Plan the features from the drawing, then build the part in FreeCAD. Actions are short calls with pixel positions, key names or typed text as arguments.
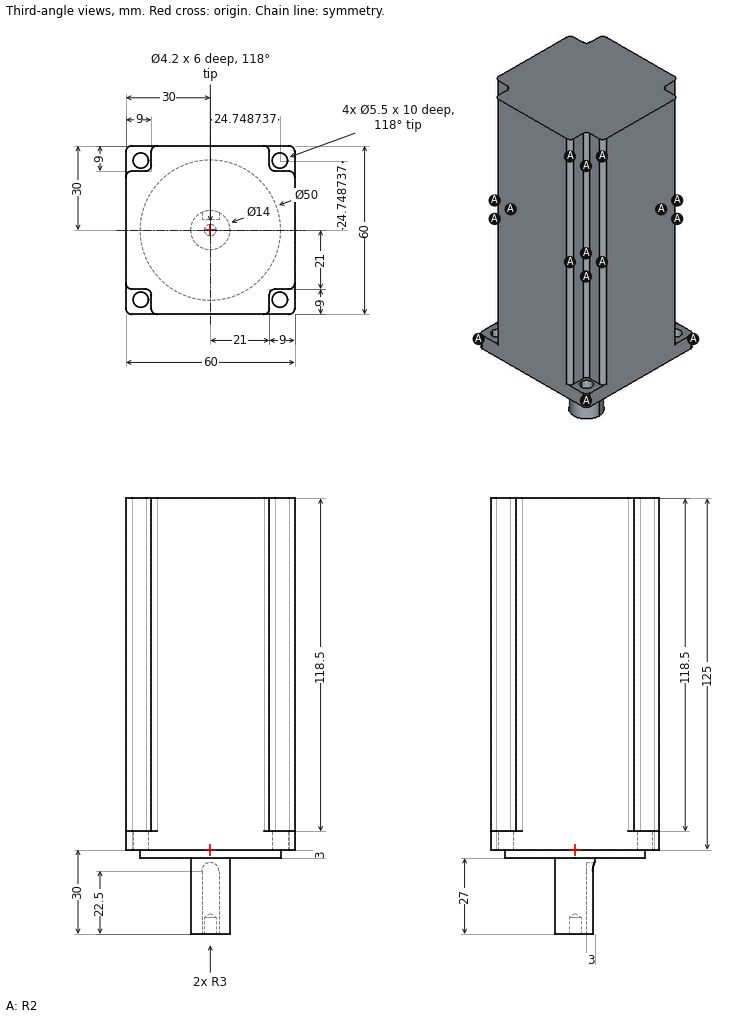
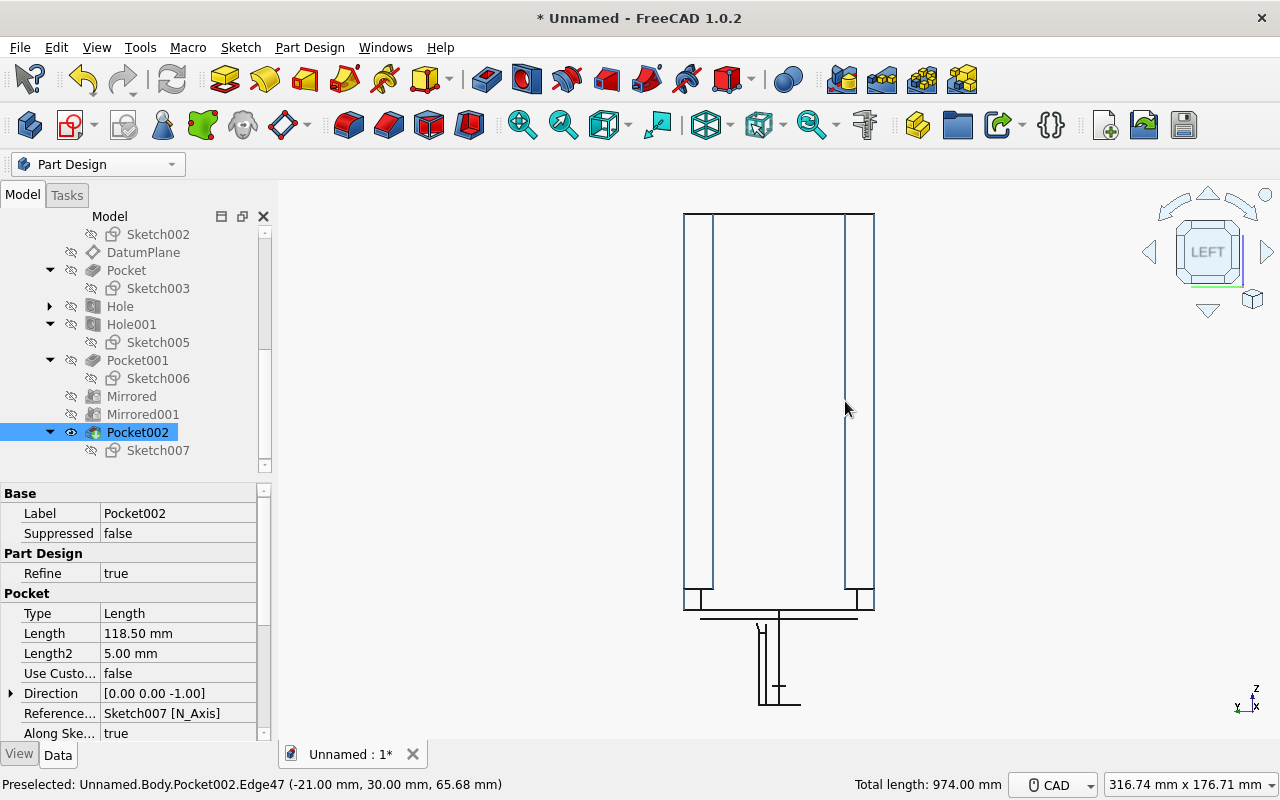
key(0)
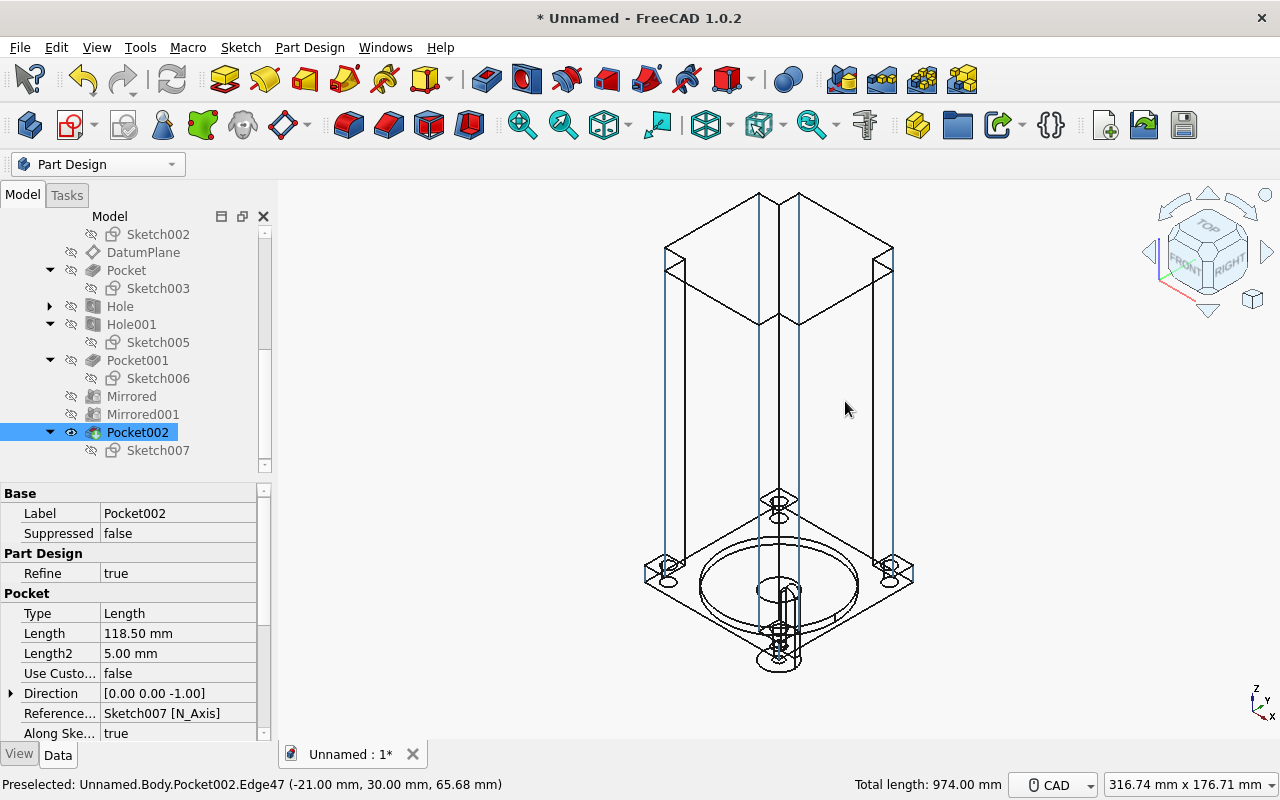
click(685, 411, ctrl)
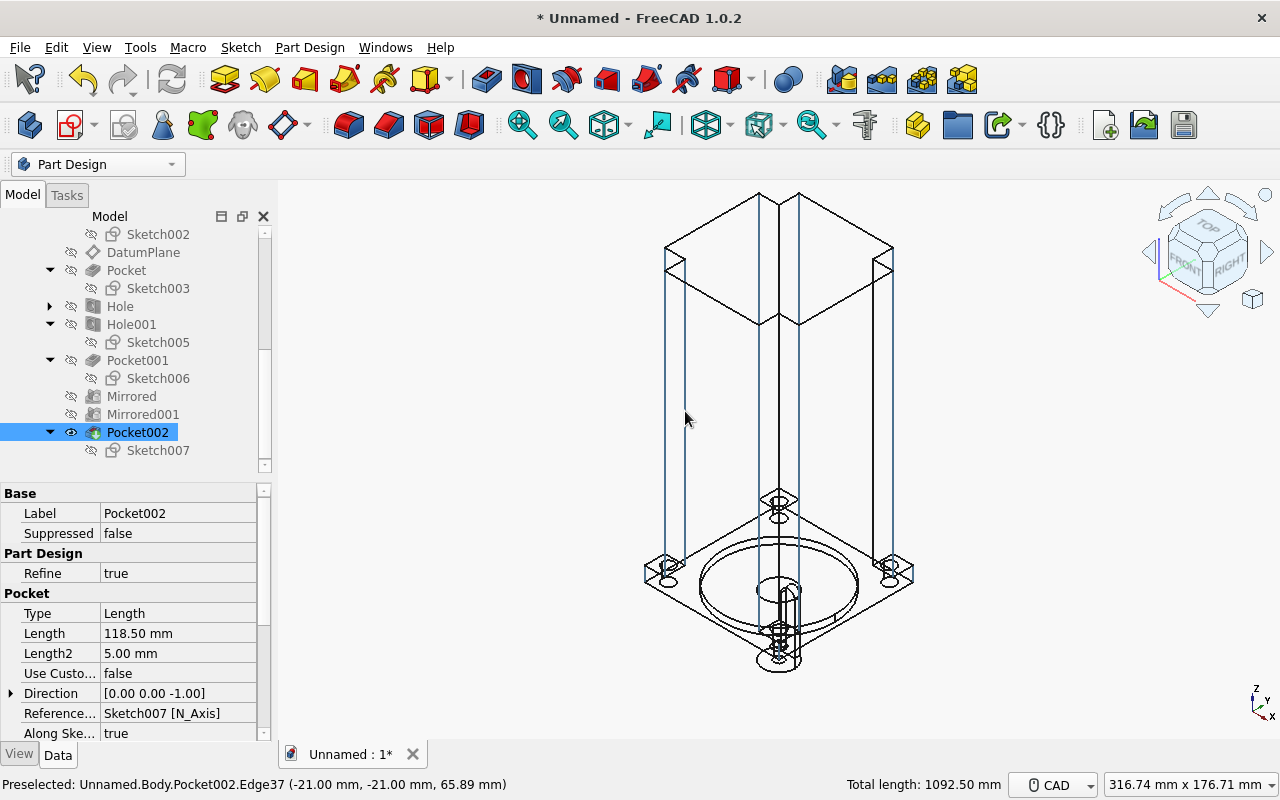
click(779, 296, ctrl)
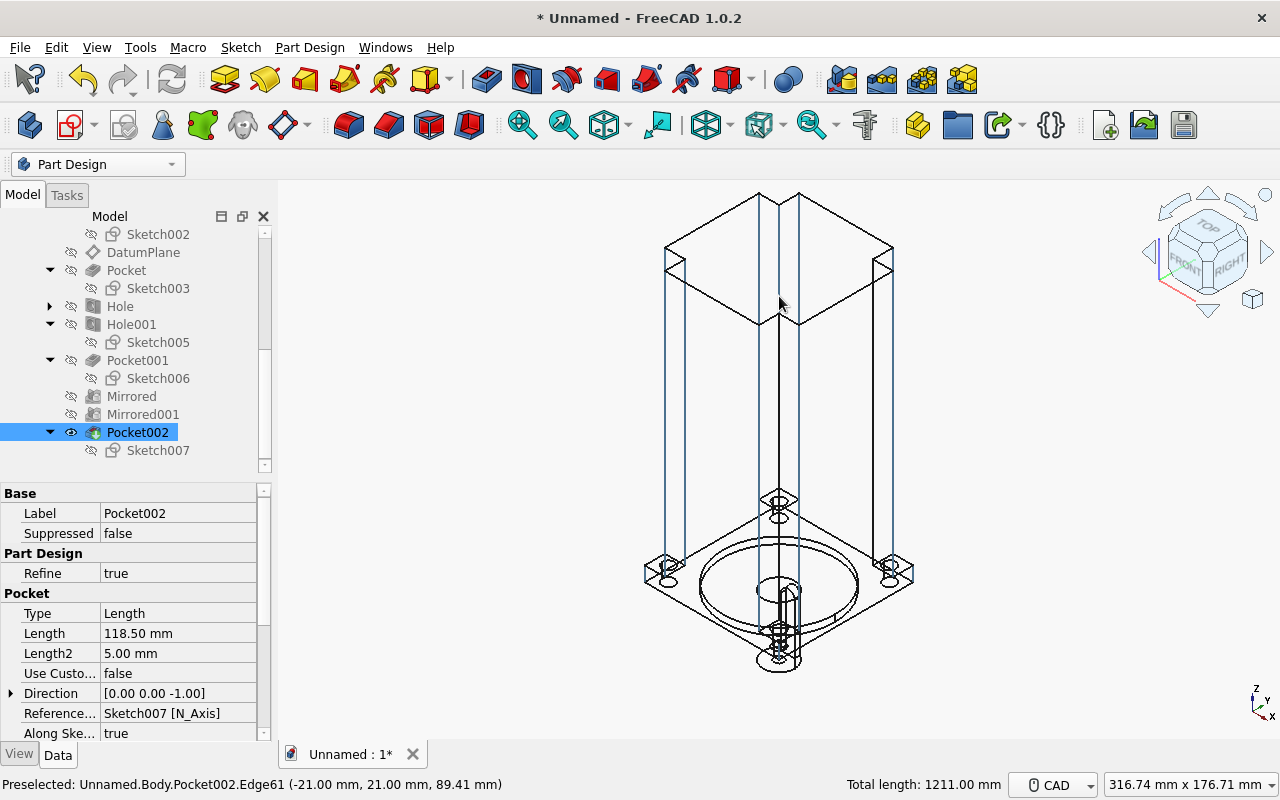
click(873, 411, ctrl)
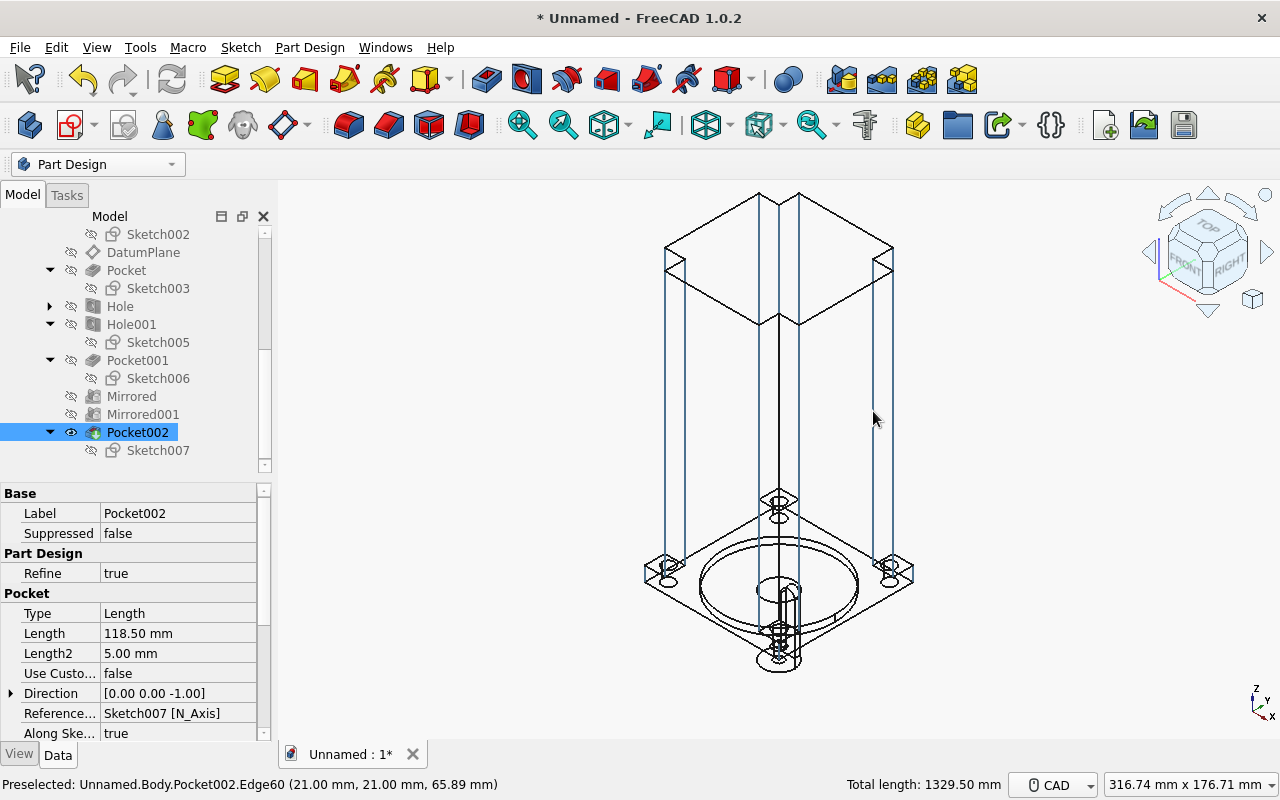
click(779, 466, ctrl)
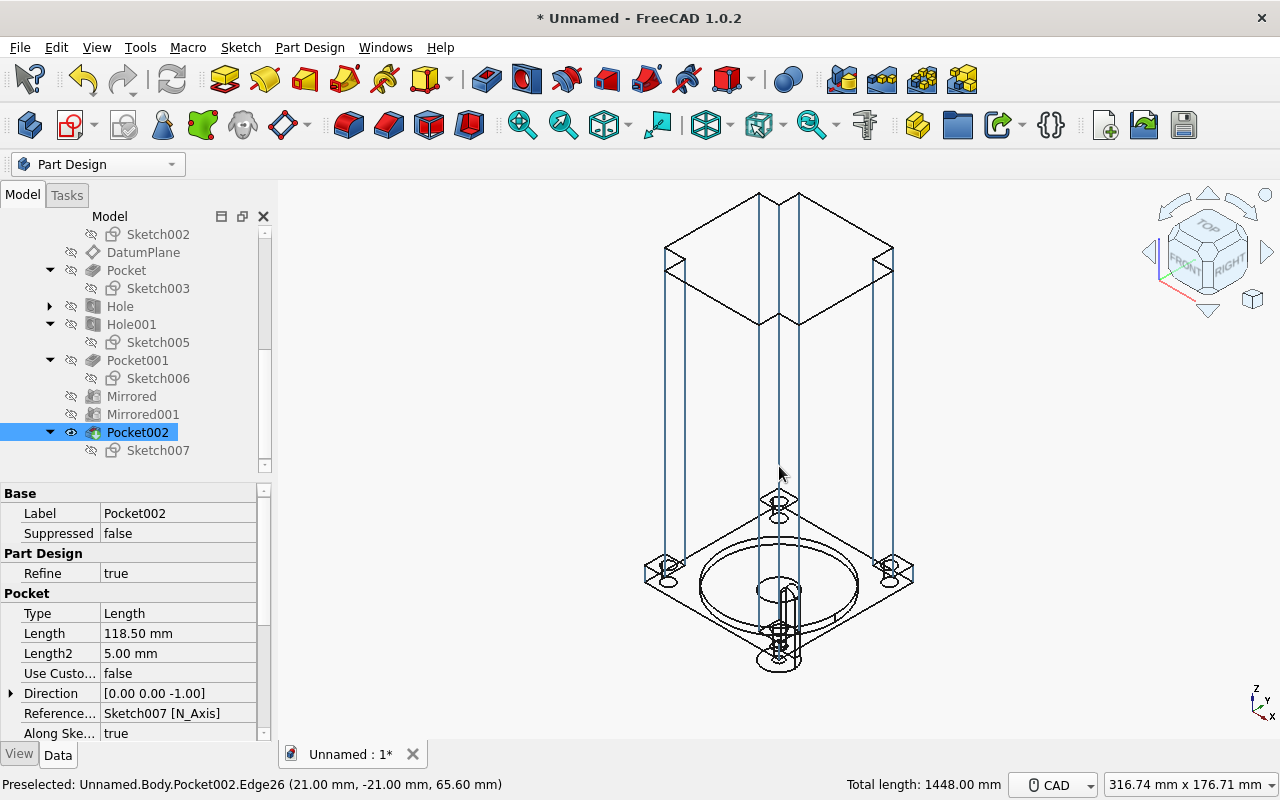
key(v)
key(1)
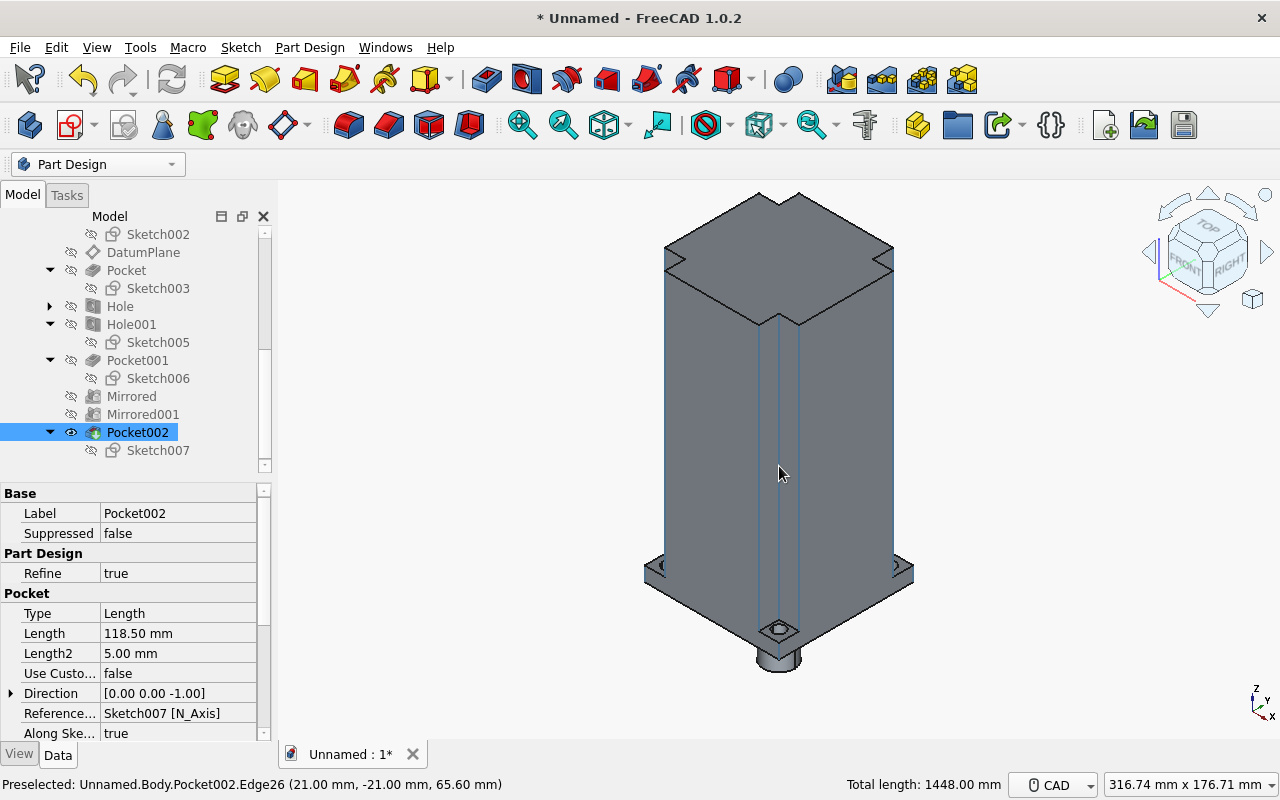
click(350, 126)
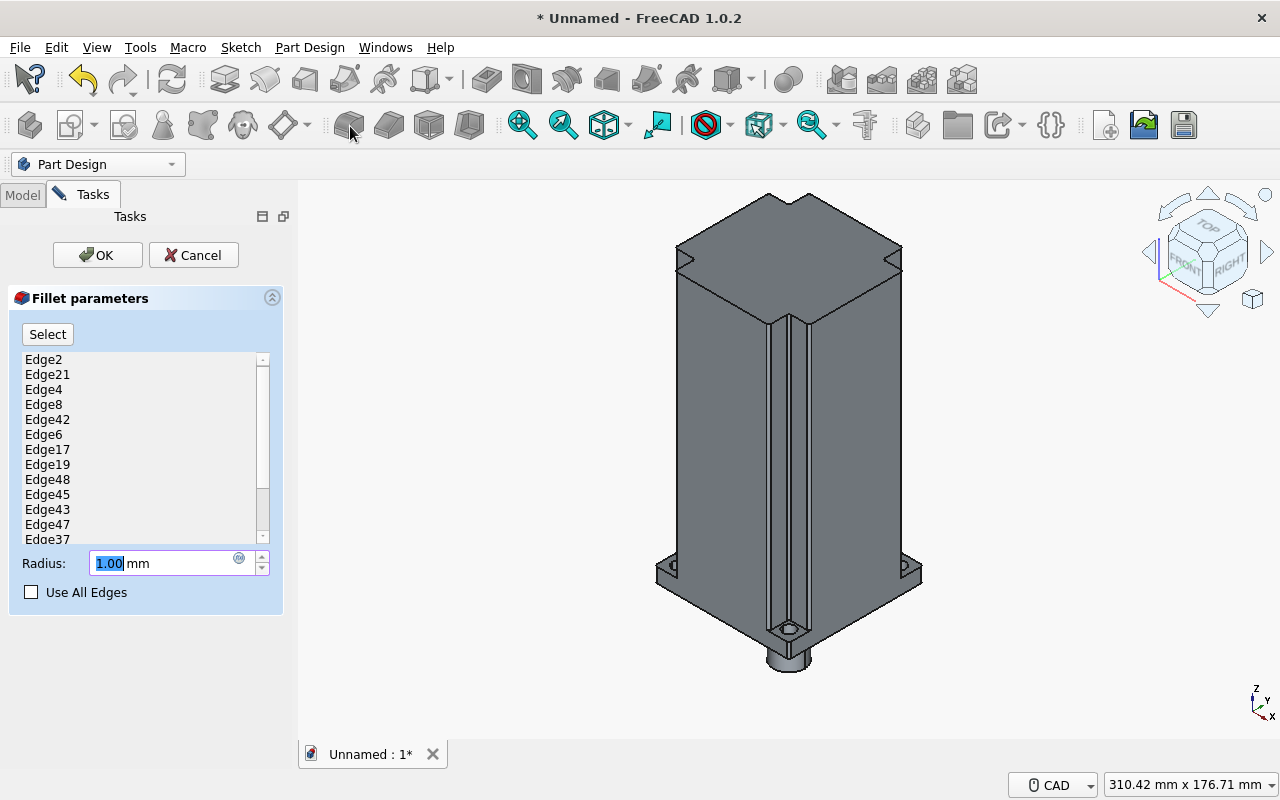
text(2)
key(Tab)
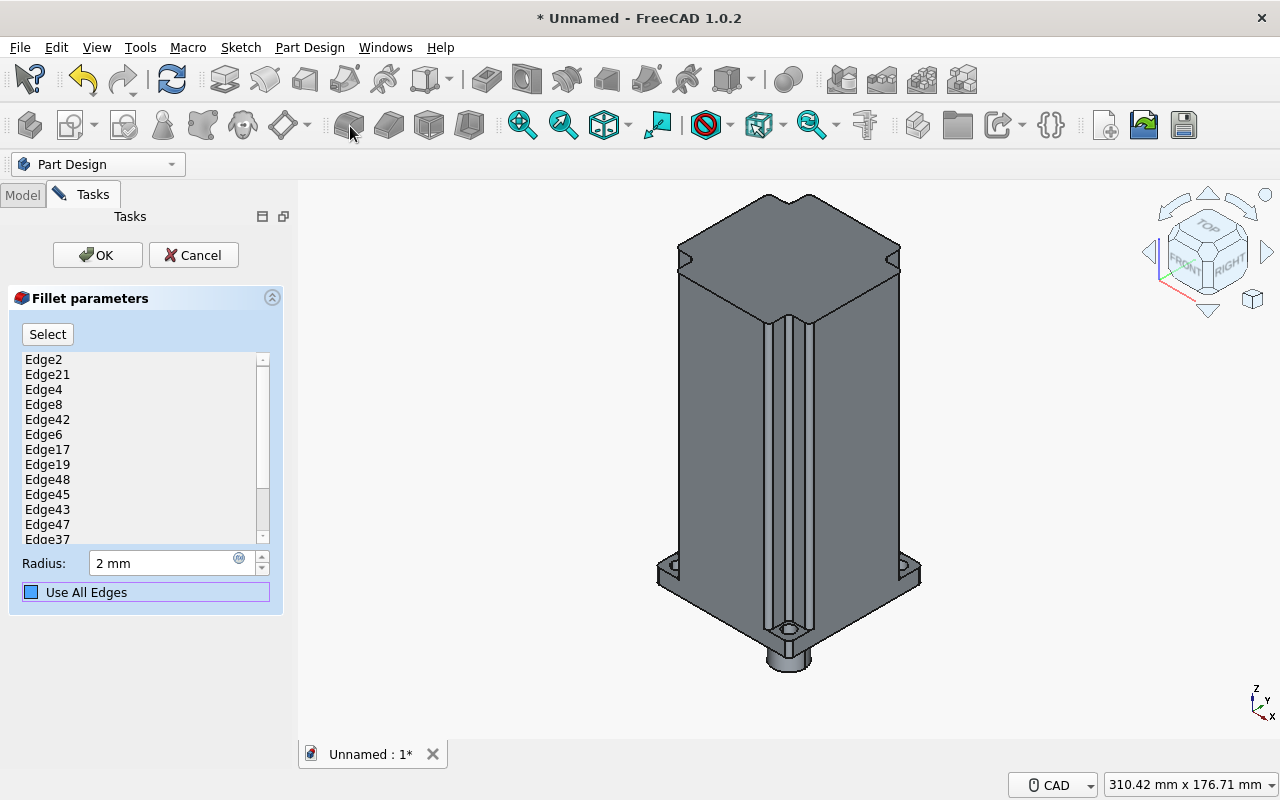
click(98, 255)